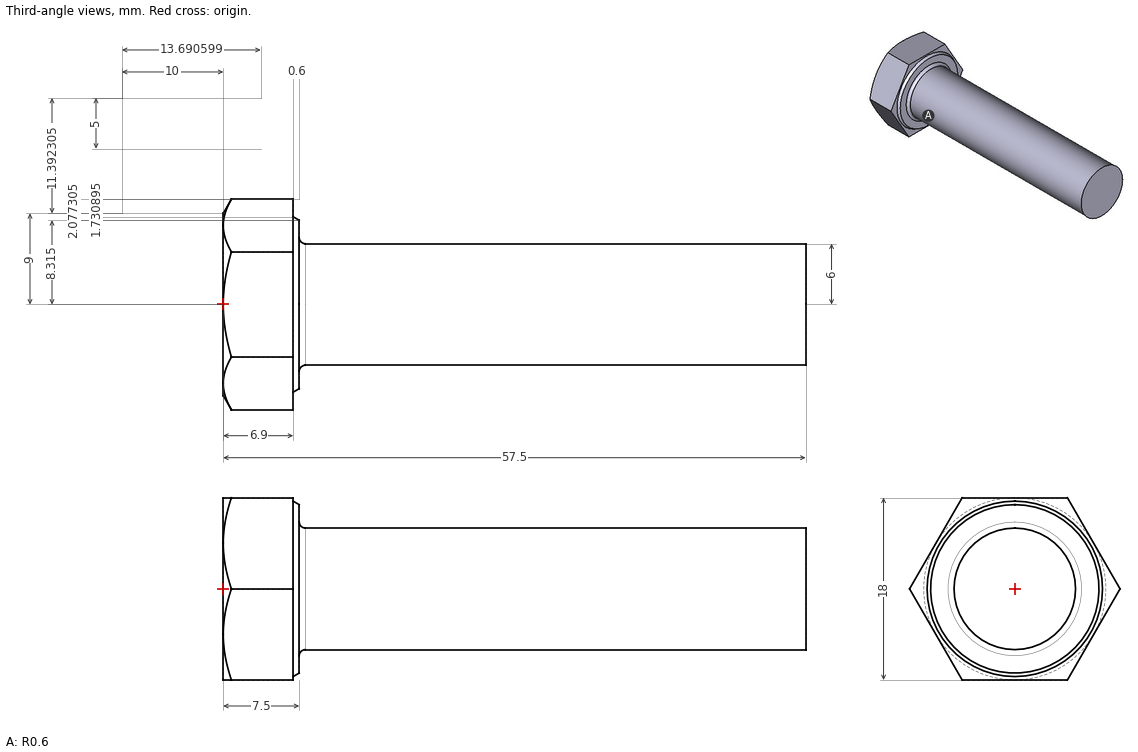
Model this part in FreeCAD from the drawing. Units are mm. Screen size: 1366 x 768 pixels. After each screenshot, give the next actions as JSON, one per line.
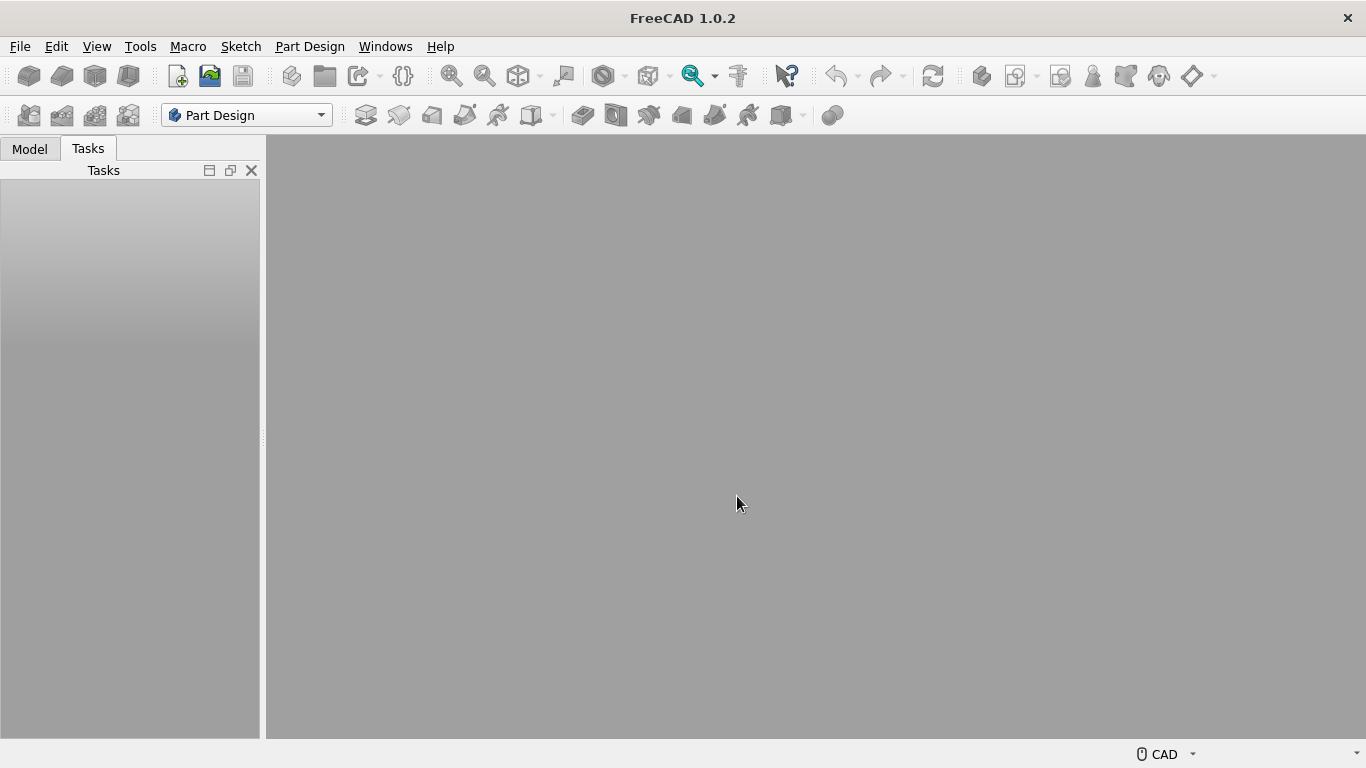
{"action": "left_click", "coordinate": [177, 76]}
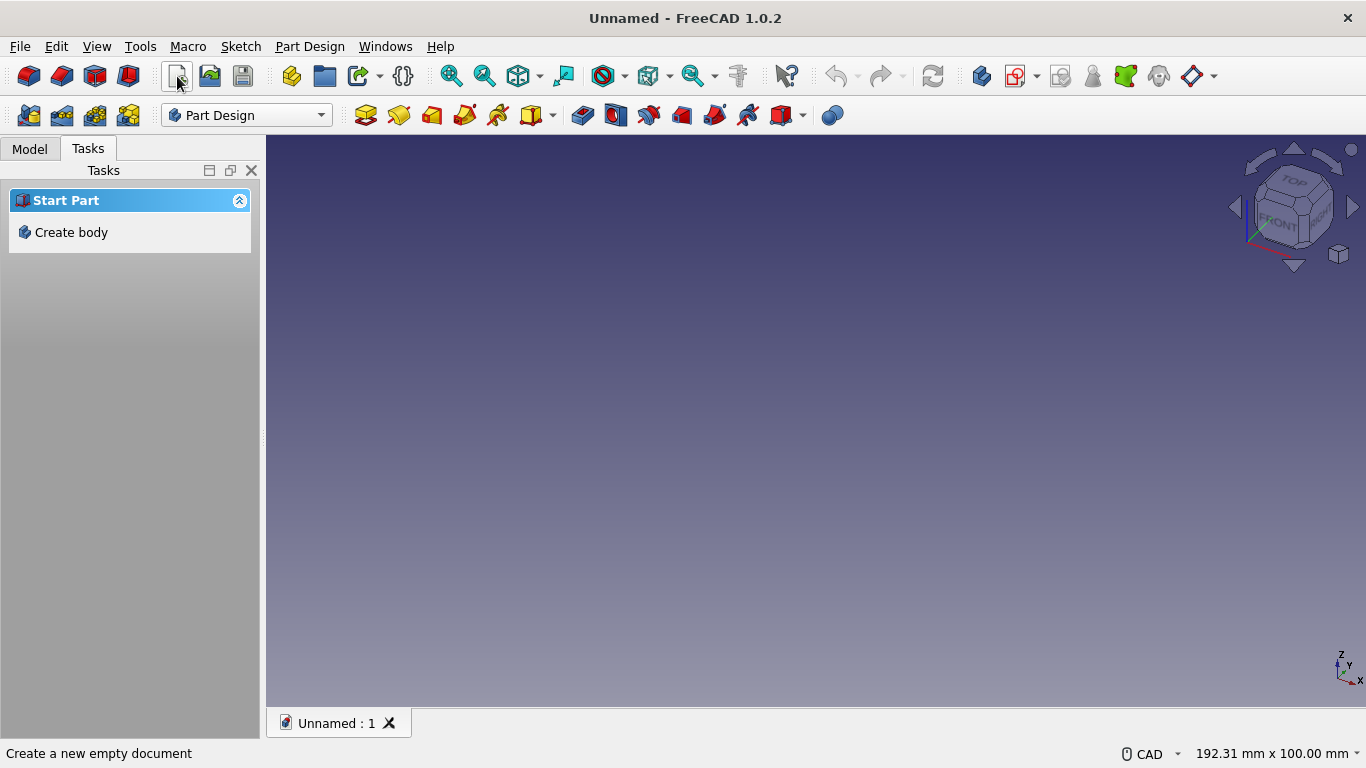
{"action": "left_click", "coordinate": [1014, 76]}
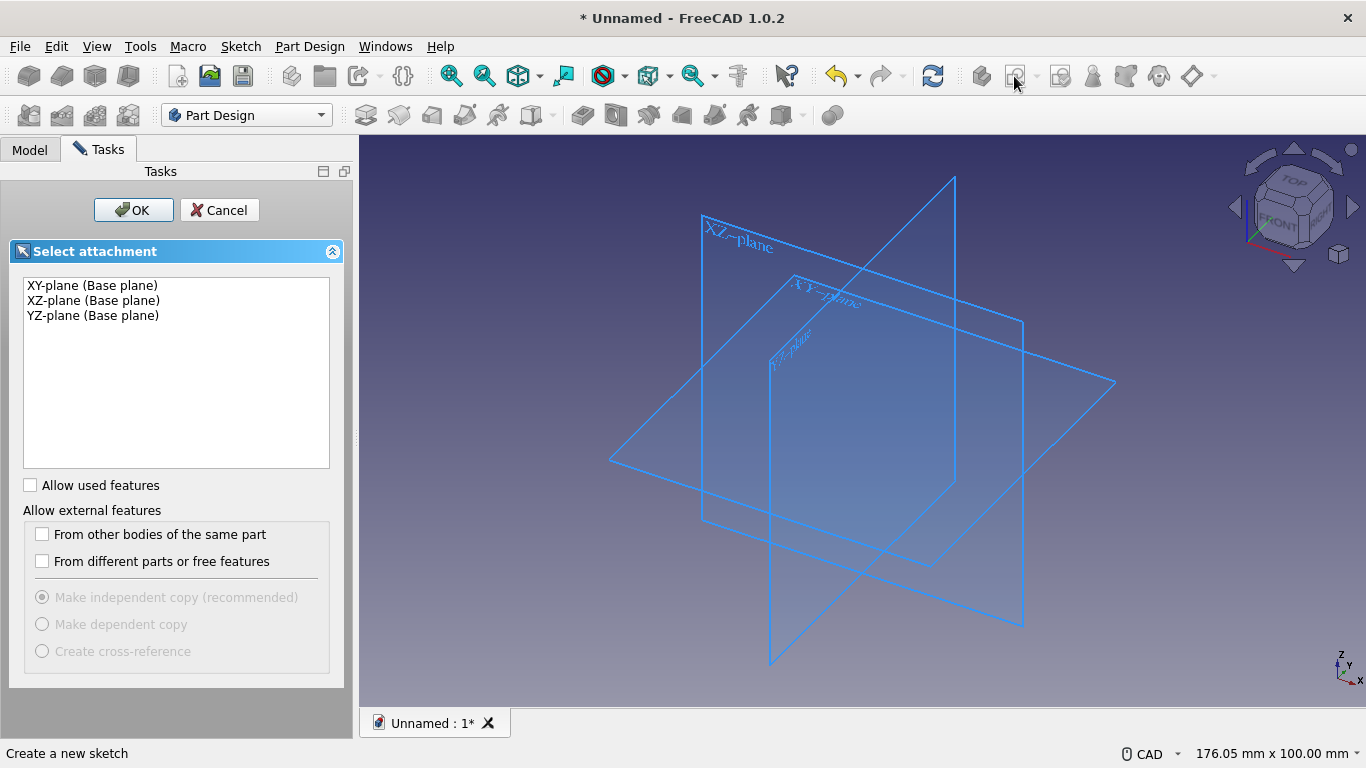
{"action": "left_click", "coordinate": [84, 316]}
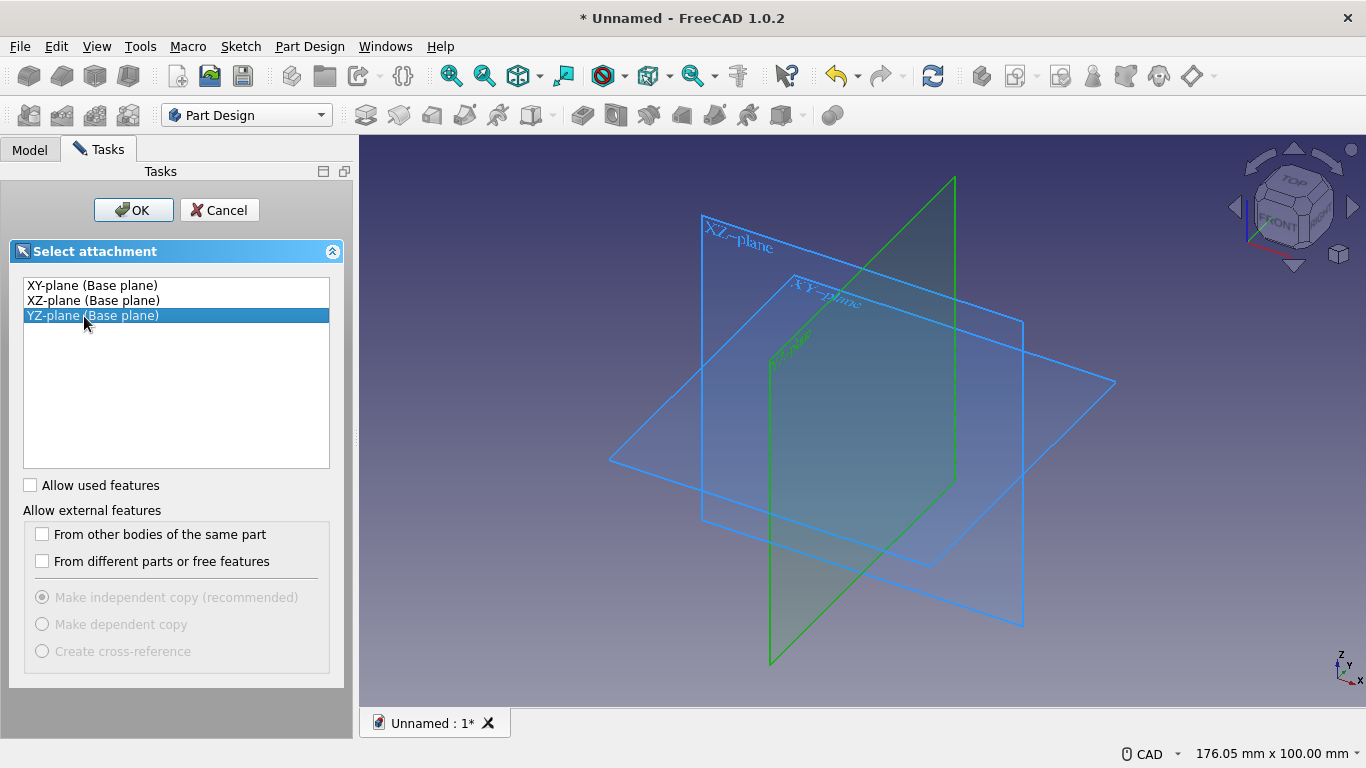
{"action": "left_click", "coordinate": [134, 210]}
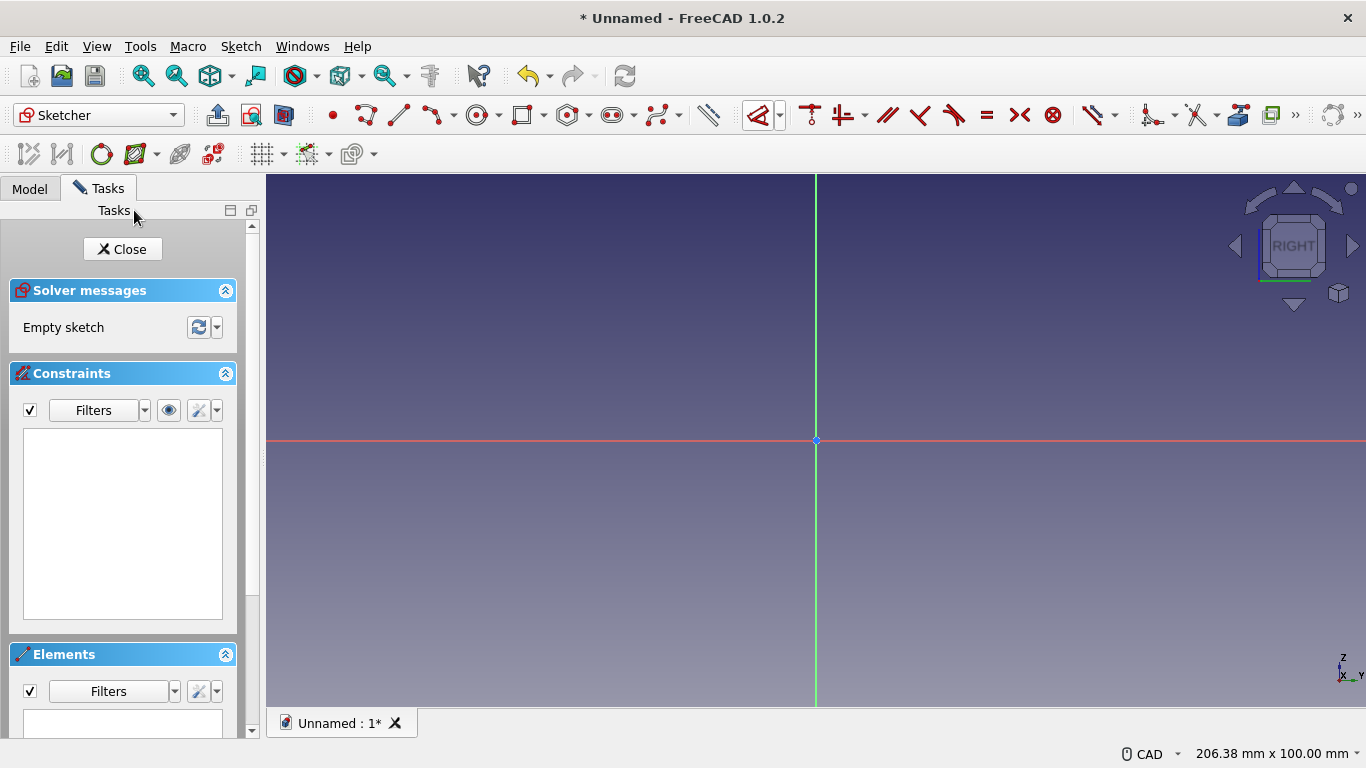
{"action": "scroll", "coordinate": [846, 440], "scroll_direction": "up", "scroll_amount": 6}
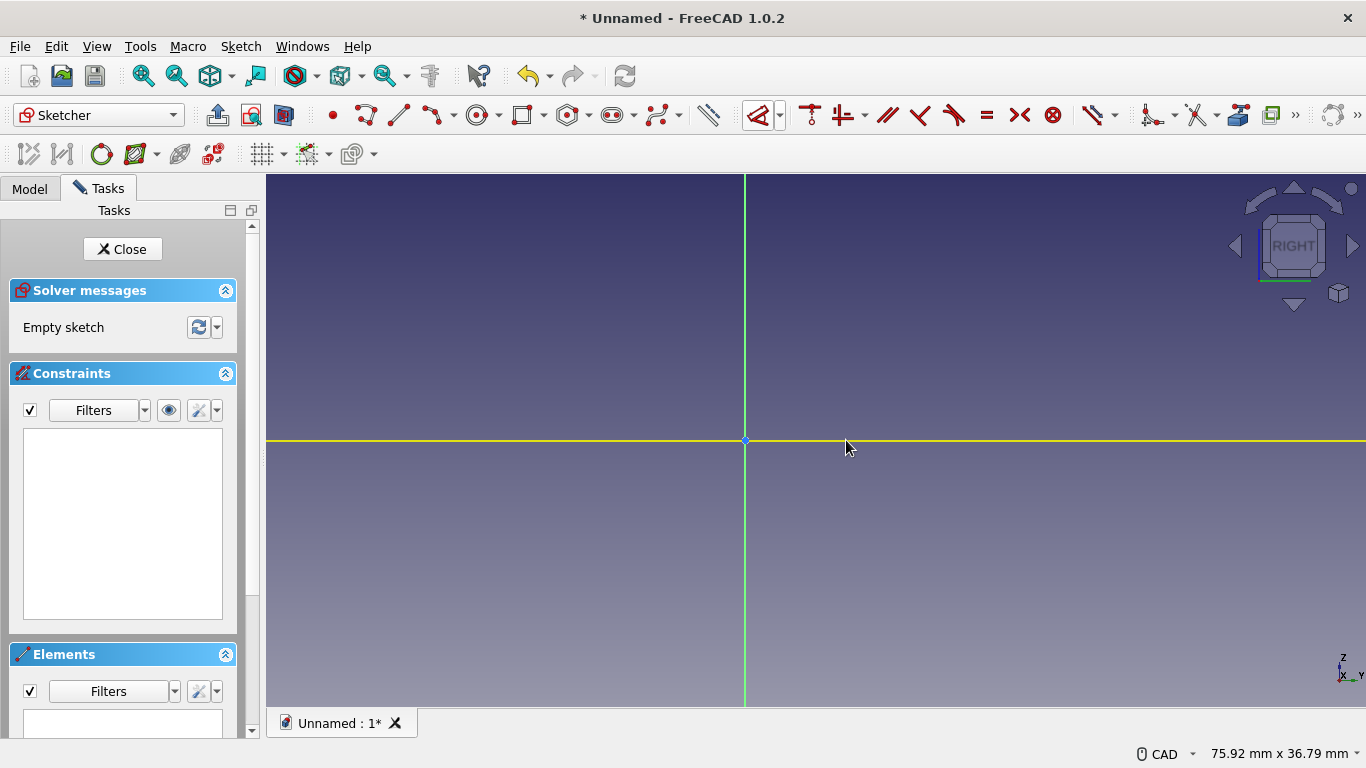
{"action": "left_click", "coordinate": [566, 116]}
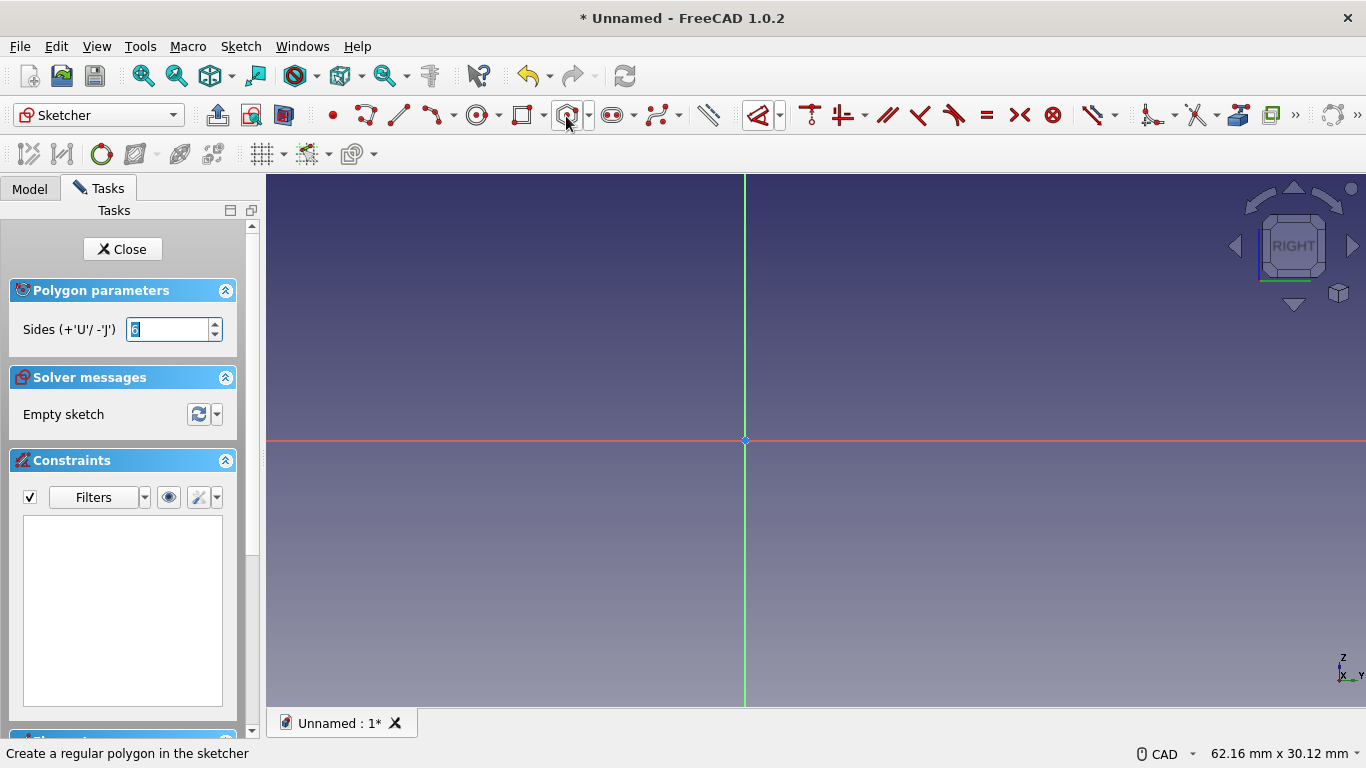
{"action": "left_click", "coordinate": [745, 440]}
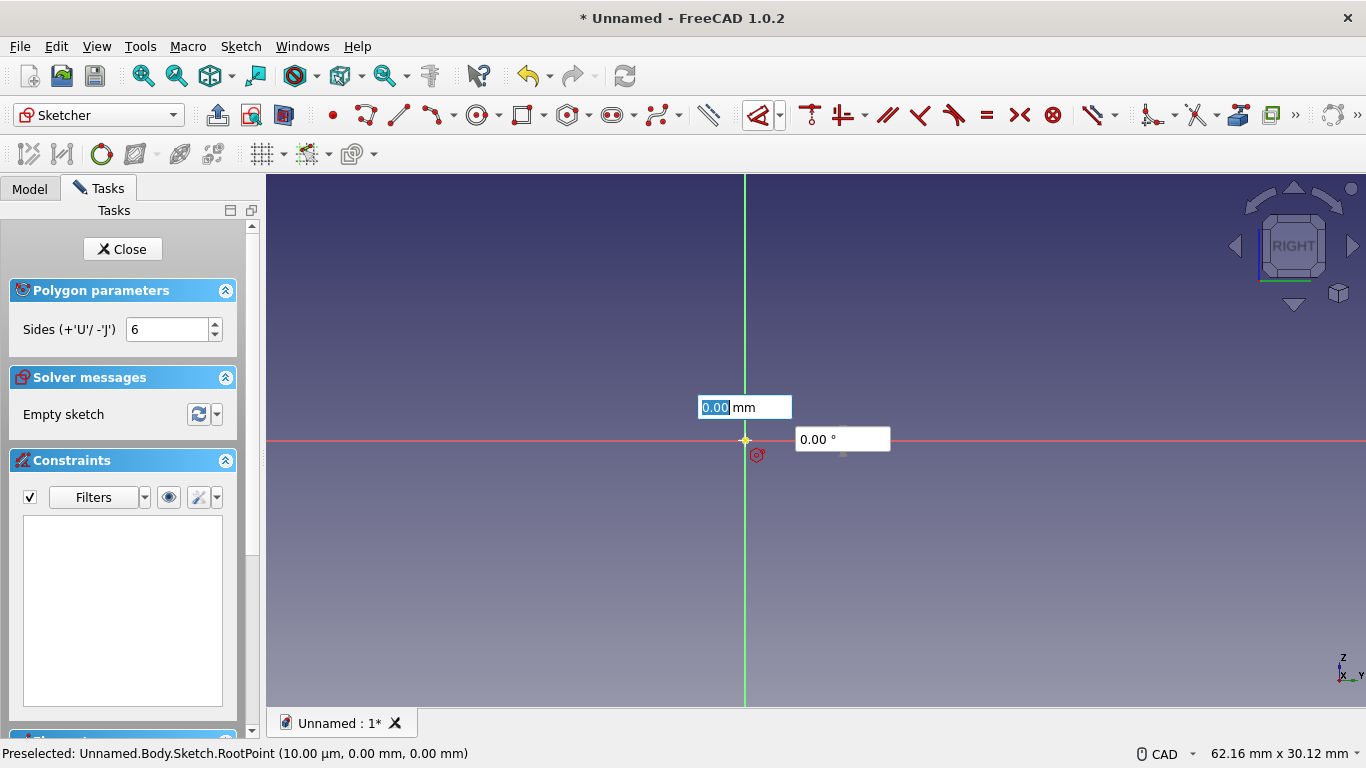
{"action": "left_click", "coordinate": [929, 440]}
{"action": "right_click", "coordinate": [929, 440]}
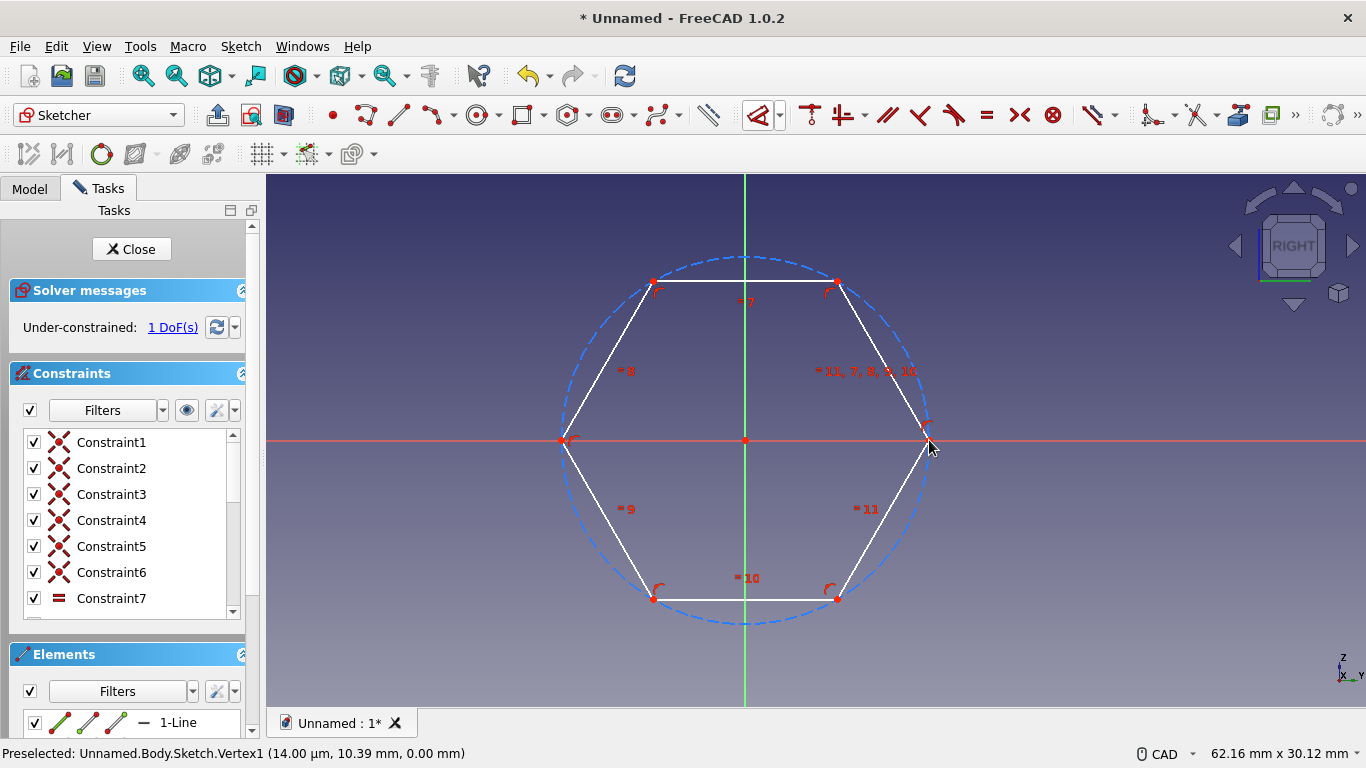
{"action": "left_click", "coordinate": [758, 116]}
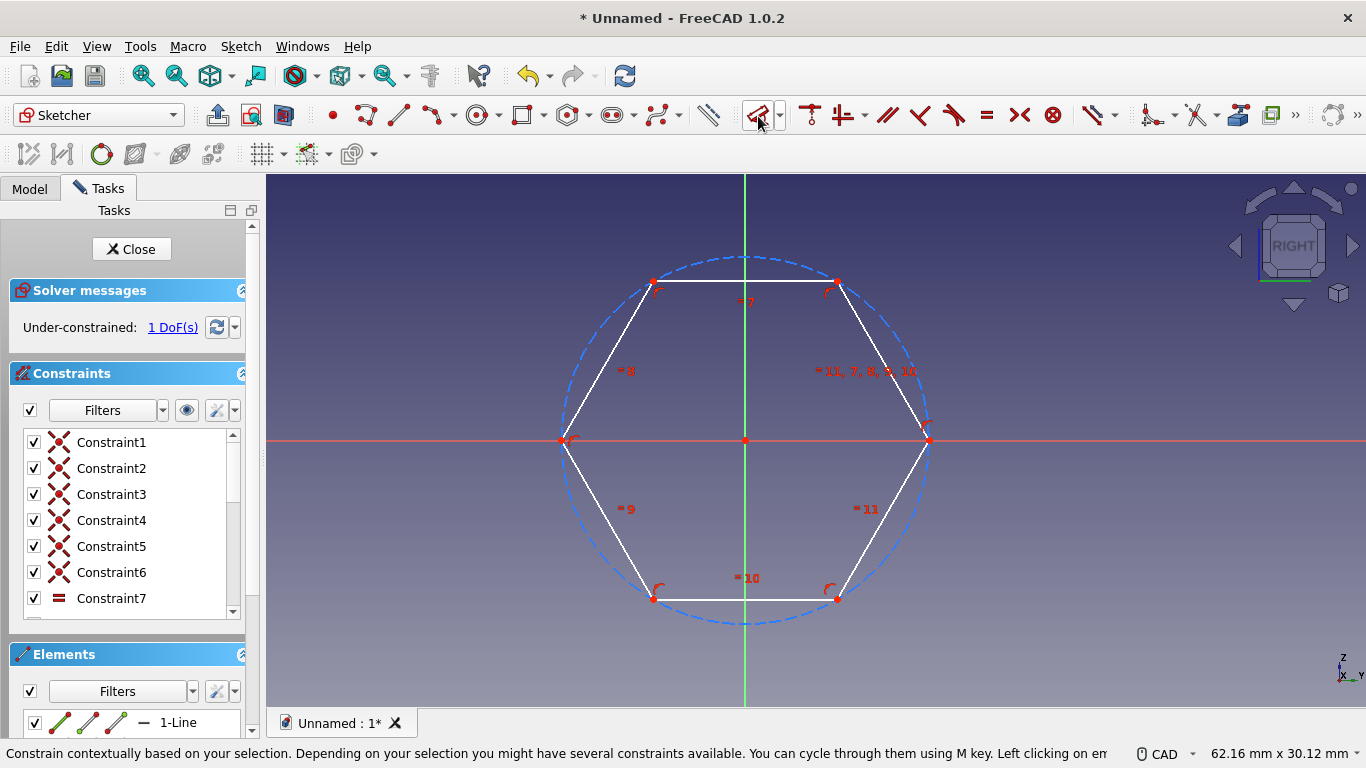
{"action": "left_click", "coordinate": [653, 600]}